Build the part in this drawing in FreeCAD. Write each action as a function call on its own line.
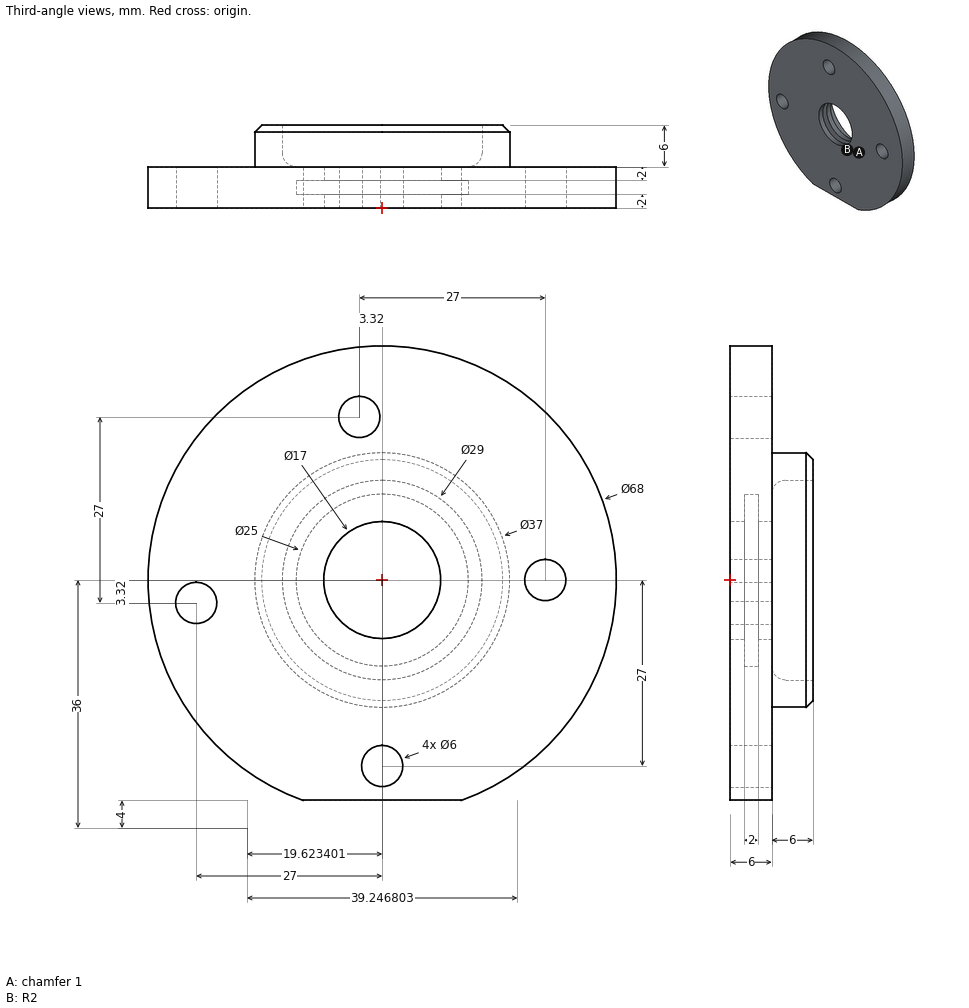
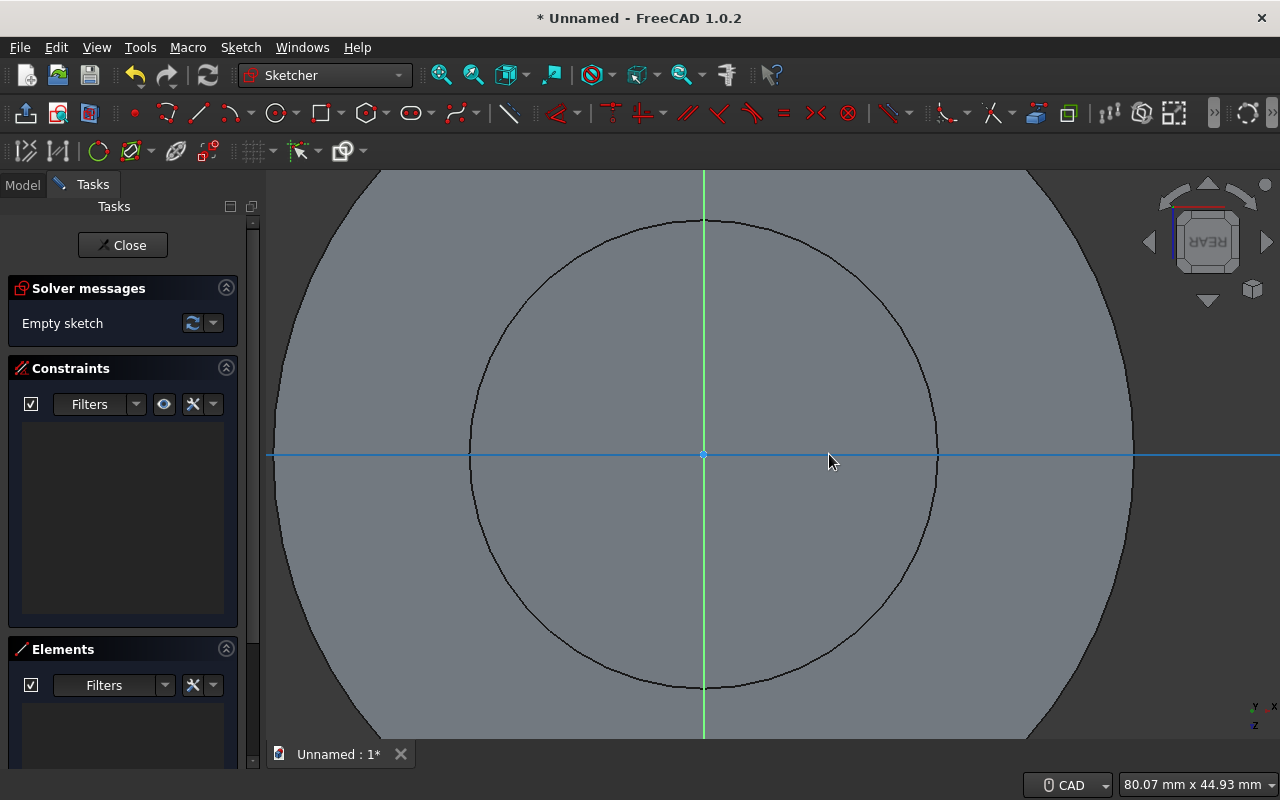
click(276, 114)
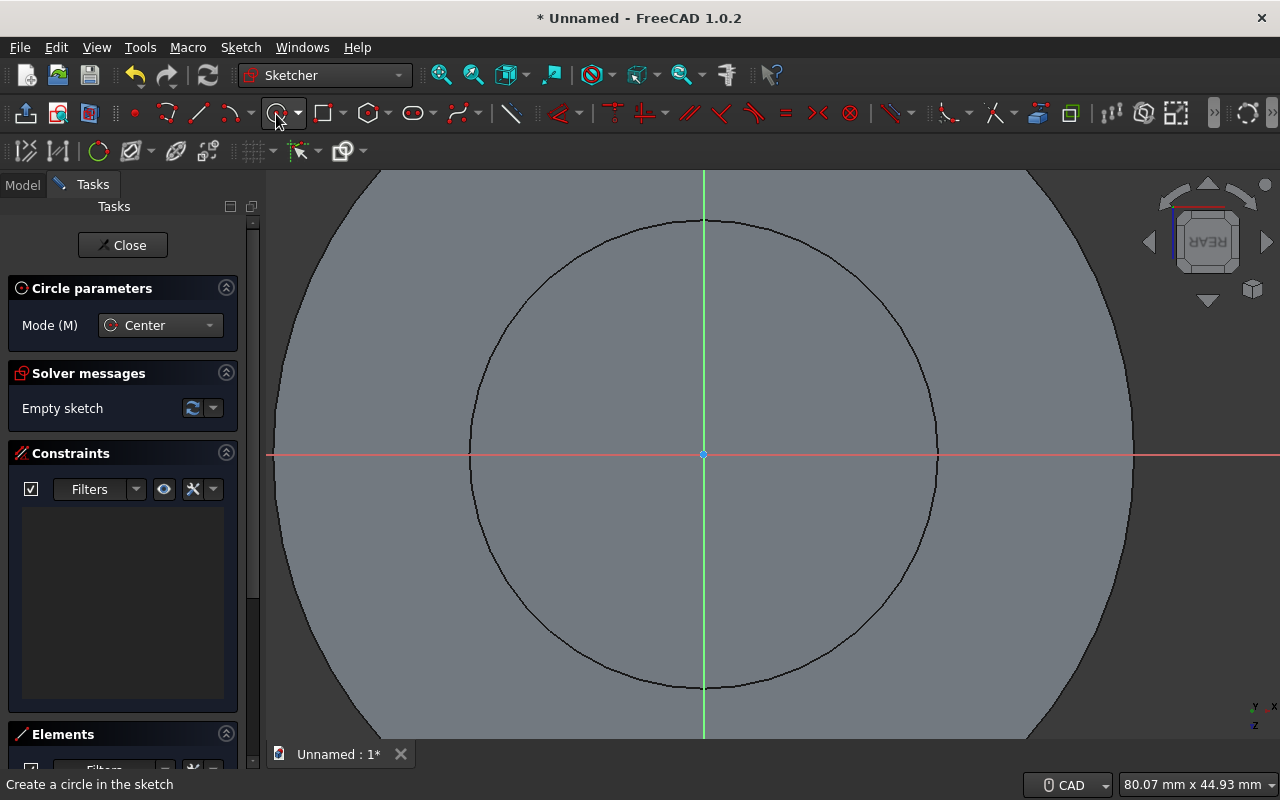
click(704, 454)
click(834, 325)
key(Escape)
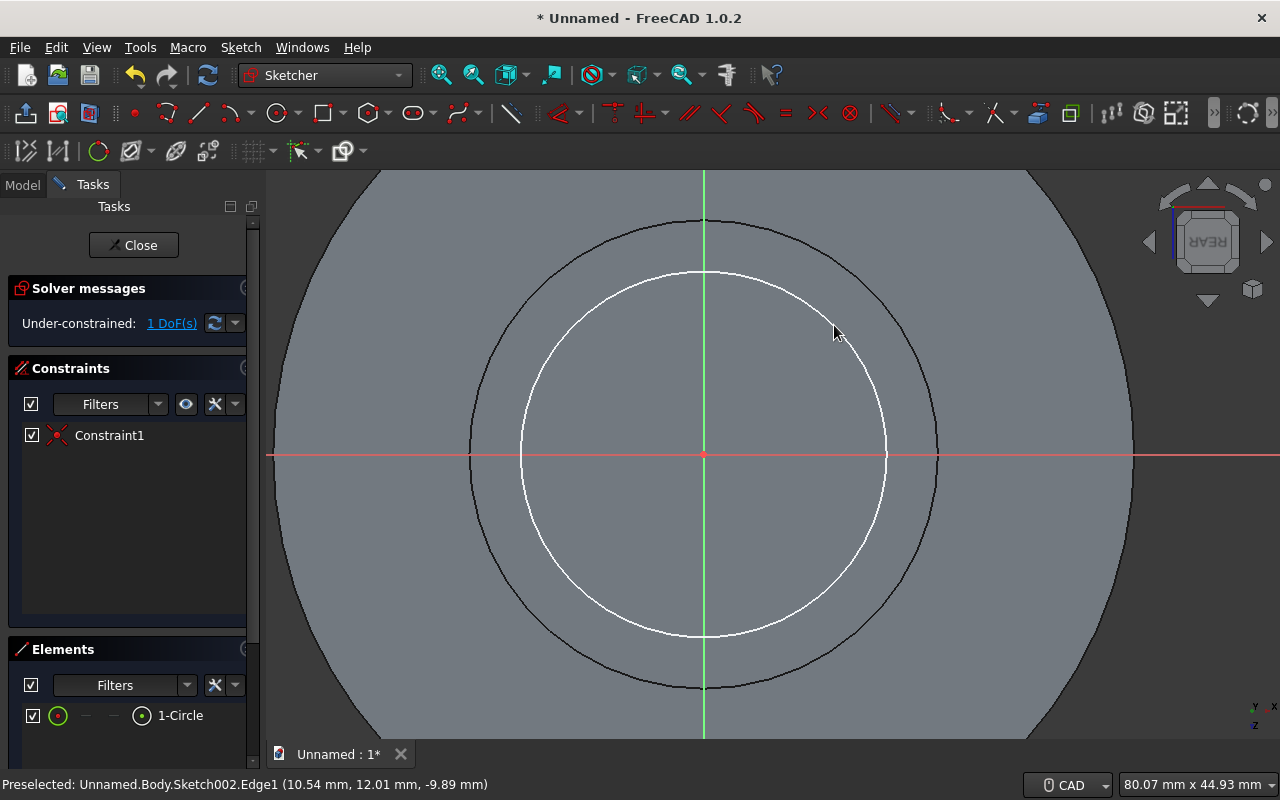
click(558, 114)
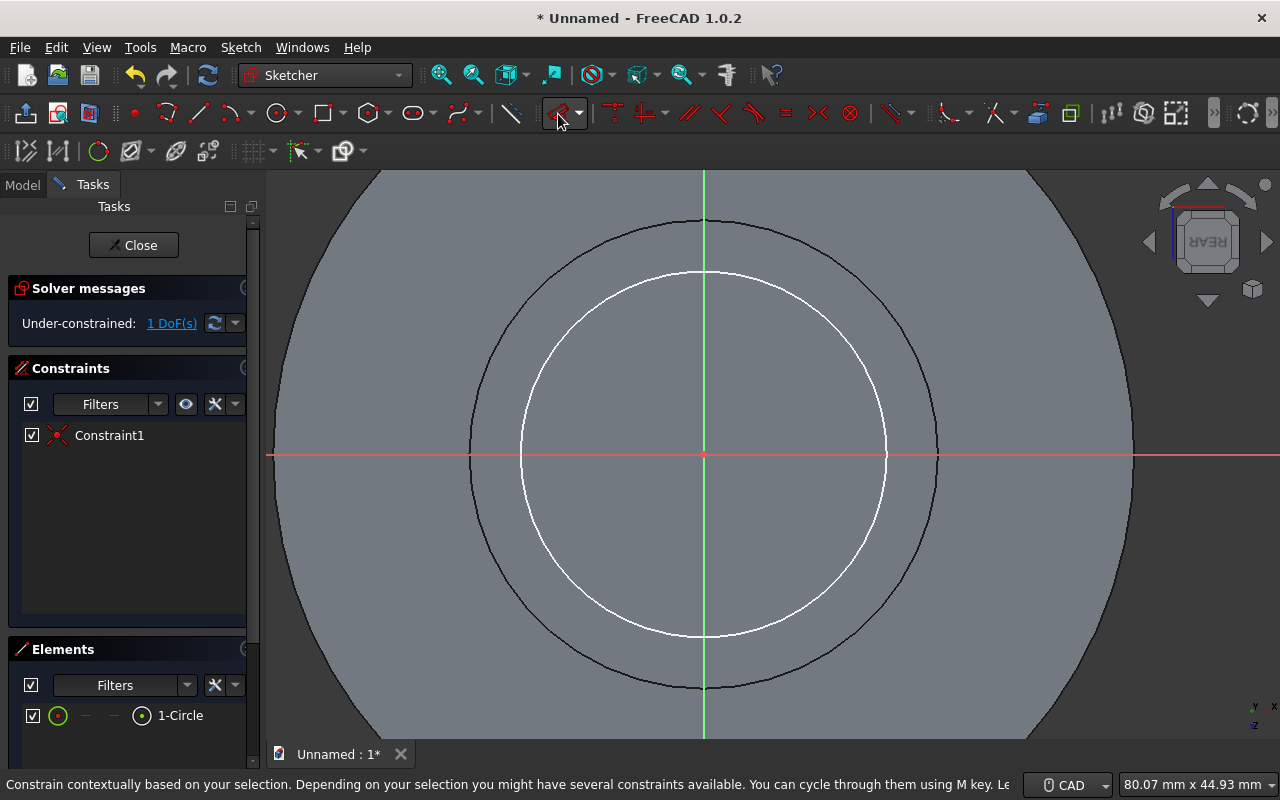
click(833, 325)
click(856, 302)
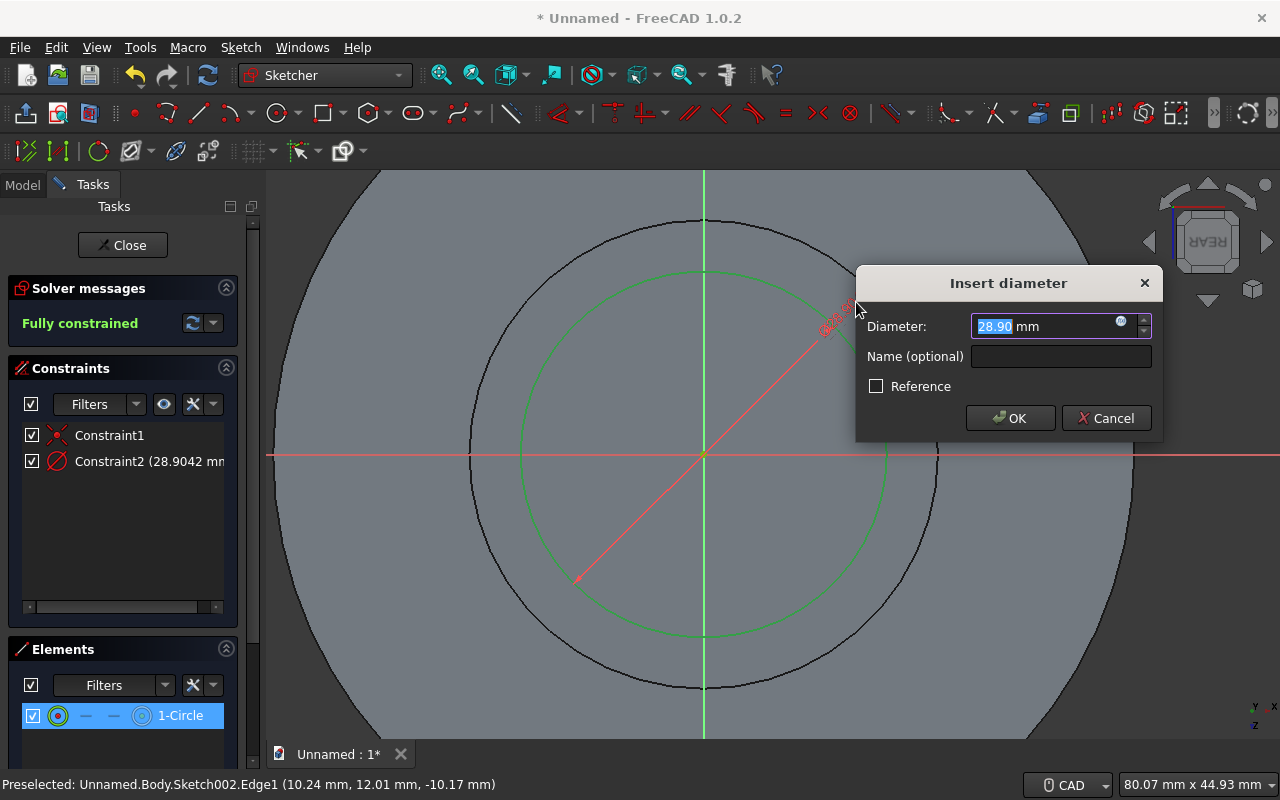
text(29)
key(Return)
key(Escape)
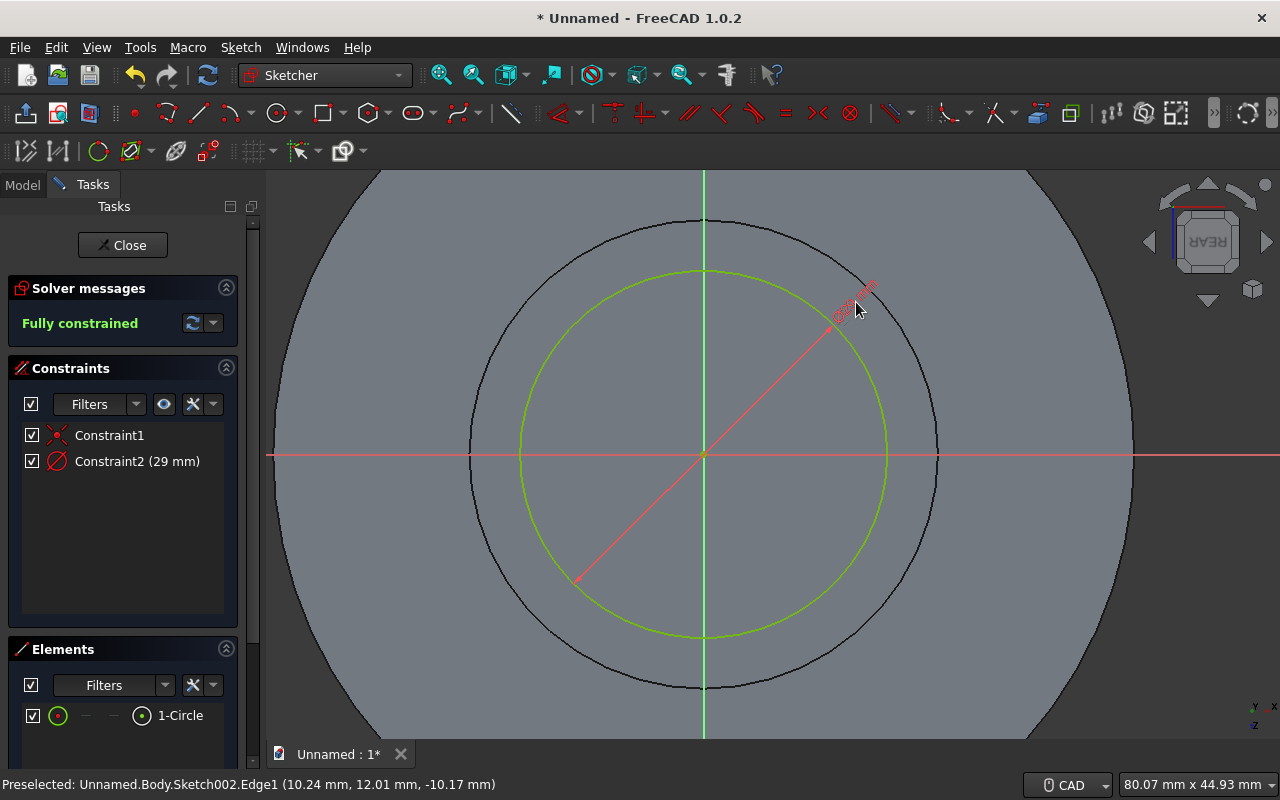
click(123, 245)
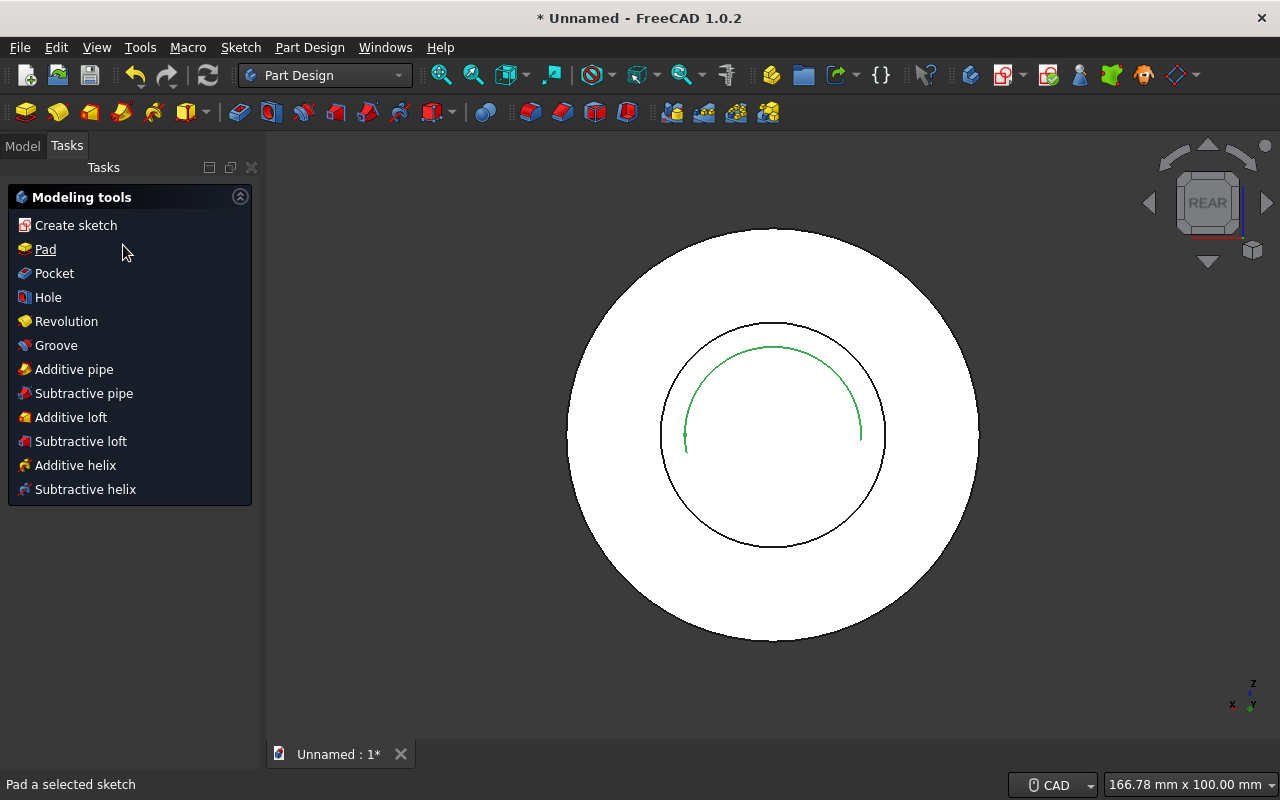
click(240, 112)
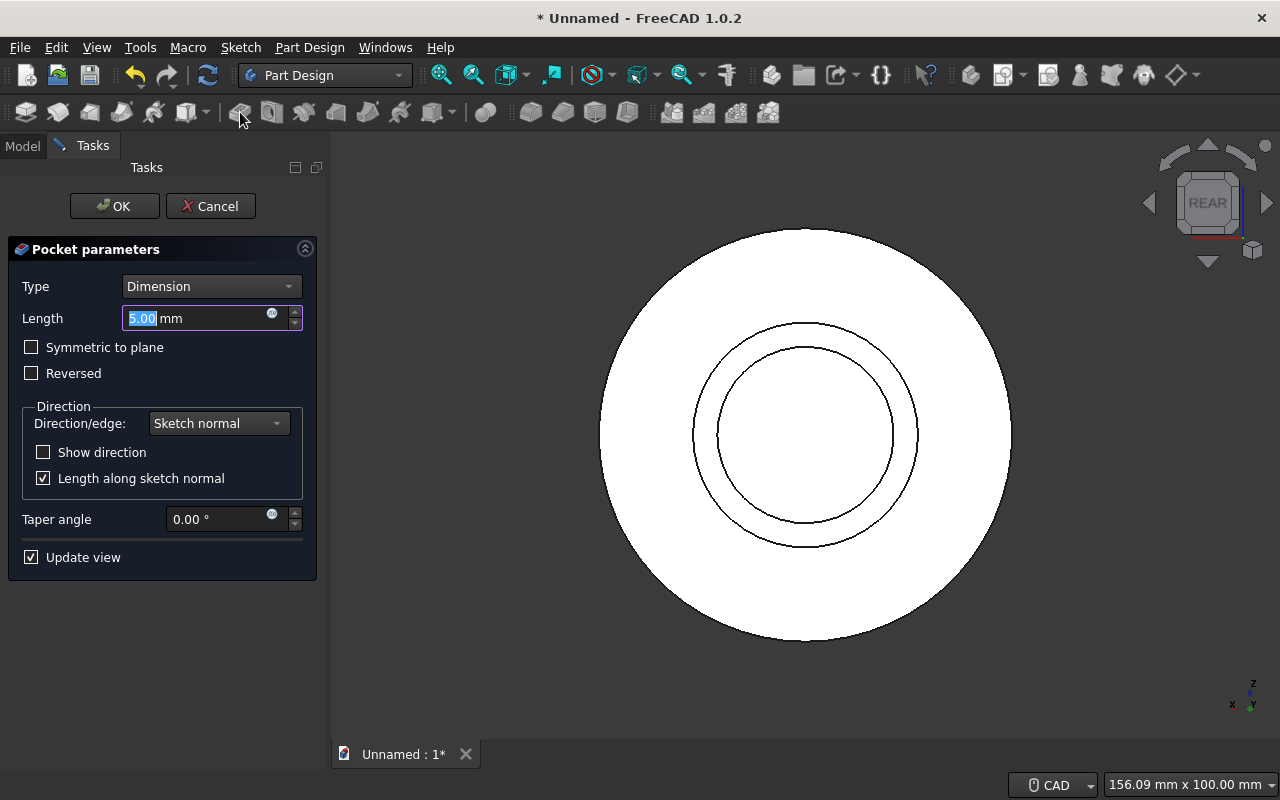
text(6)
key(Tab)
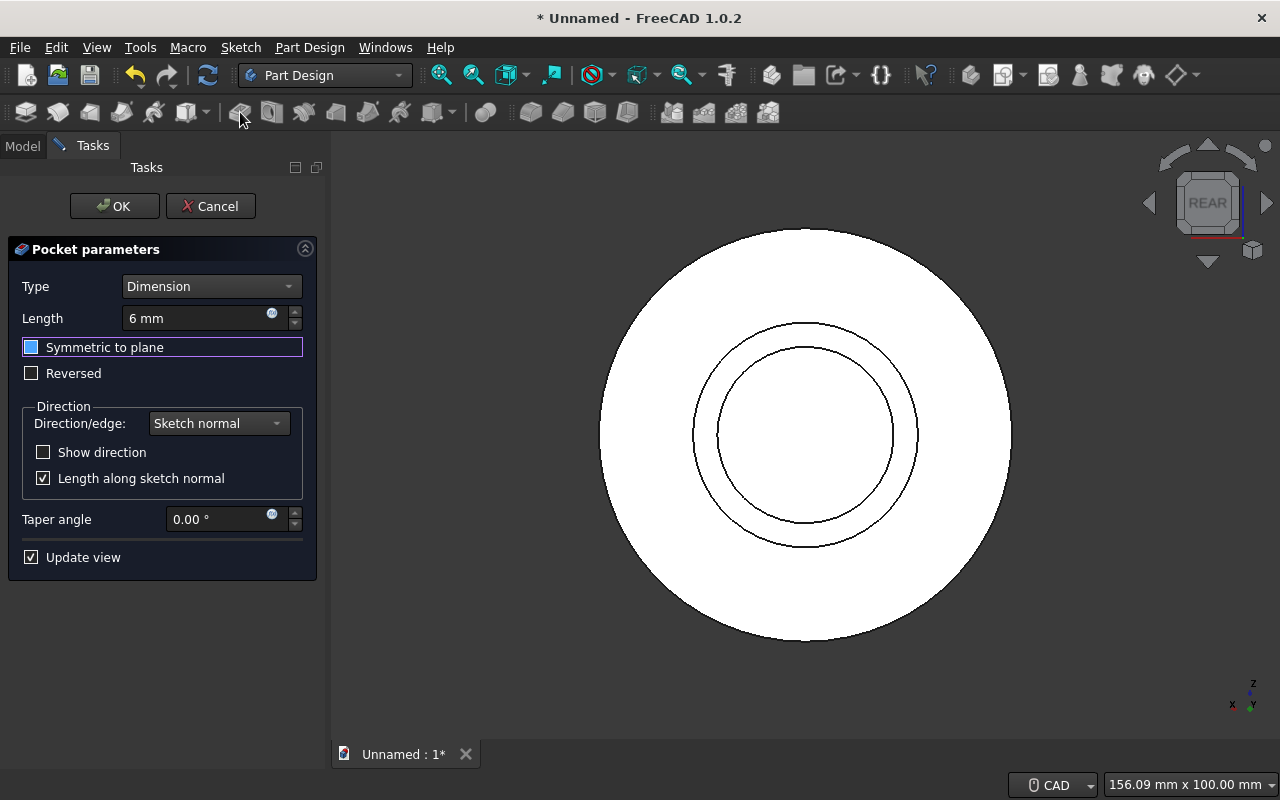
click(115, 206)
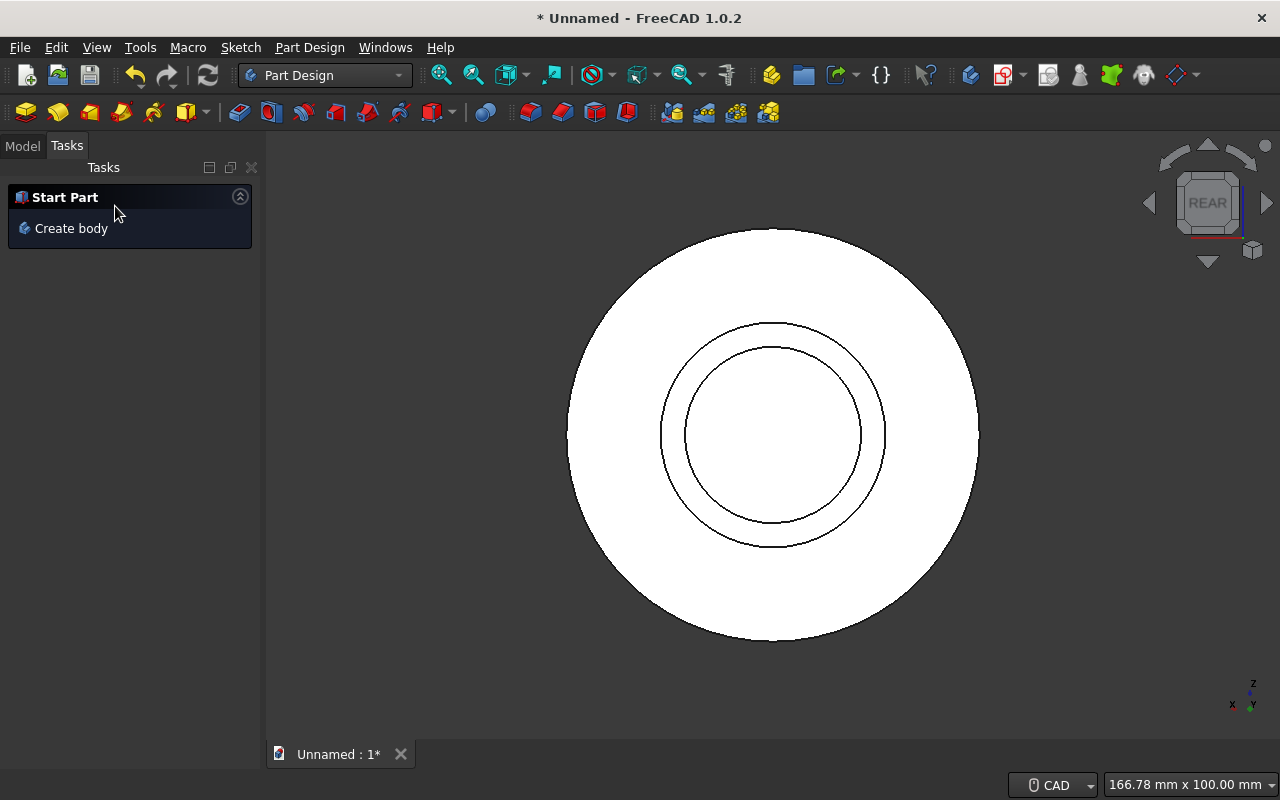
click(655, 552)